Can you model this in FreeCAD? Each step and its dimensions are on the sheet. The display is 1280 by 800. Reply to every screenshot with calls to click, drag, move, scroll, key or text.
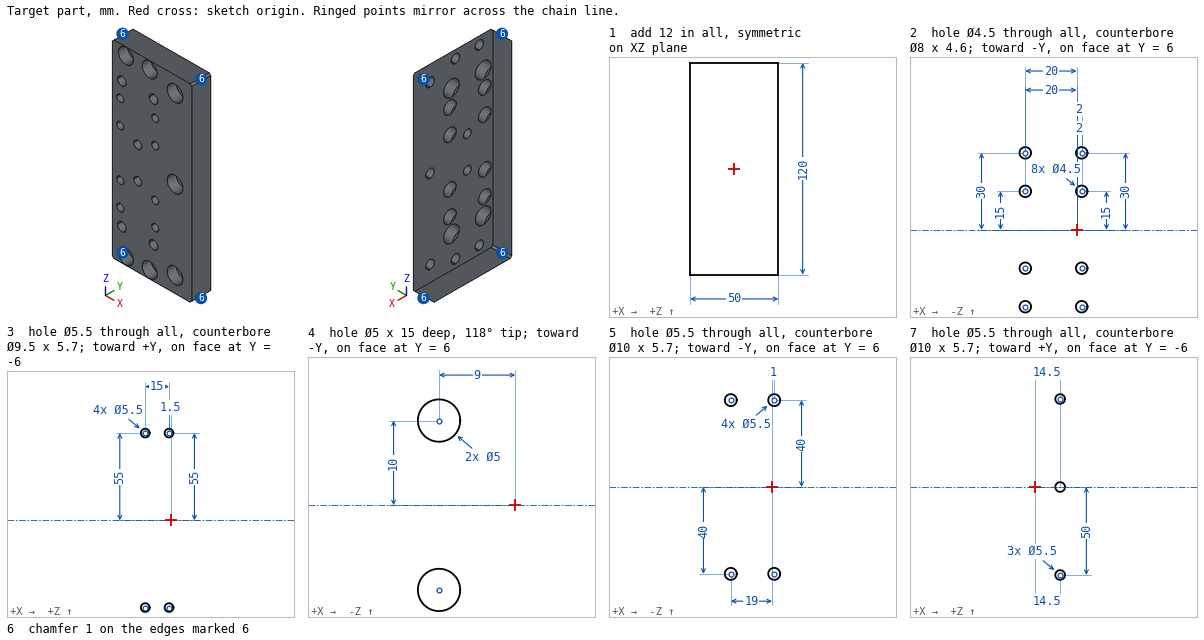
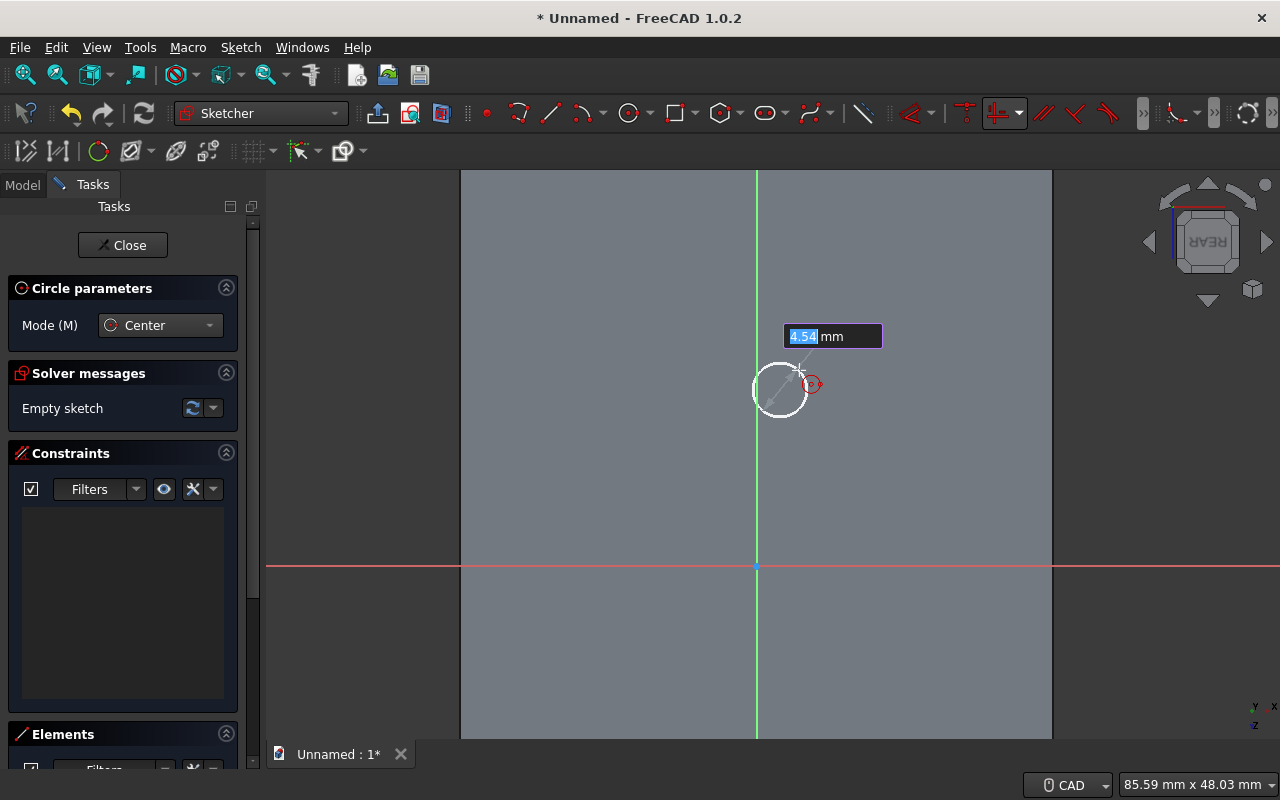
text(4.5)
key(Return)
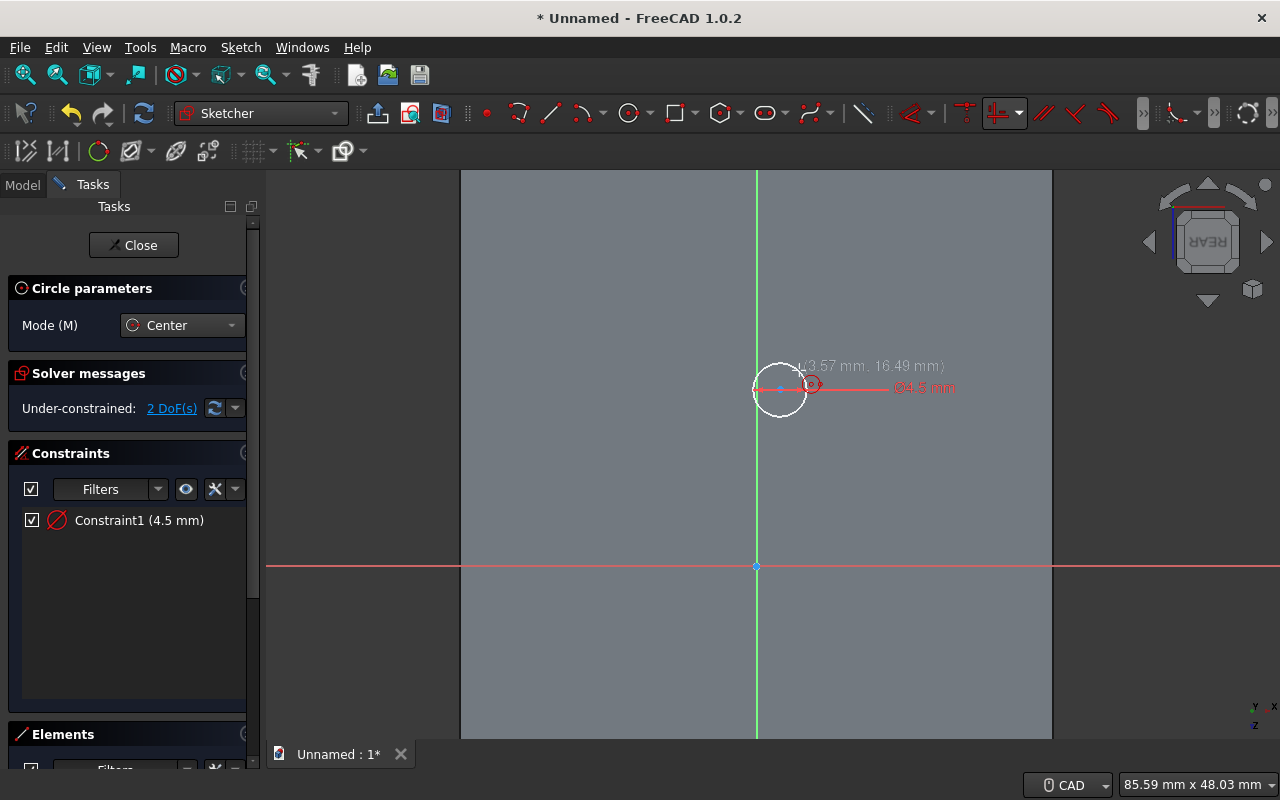
click(520, 211)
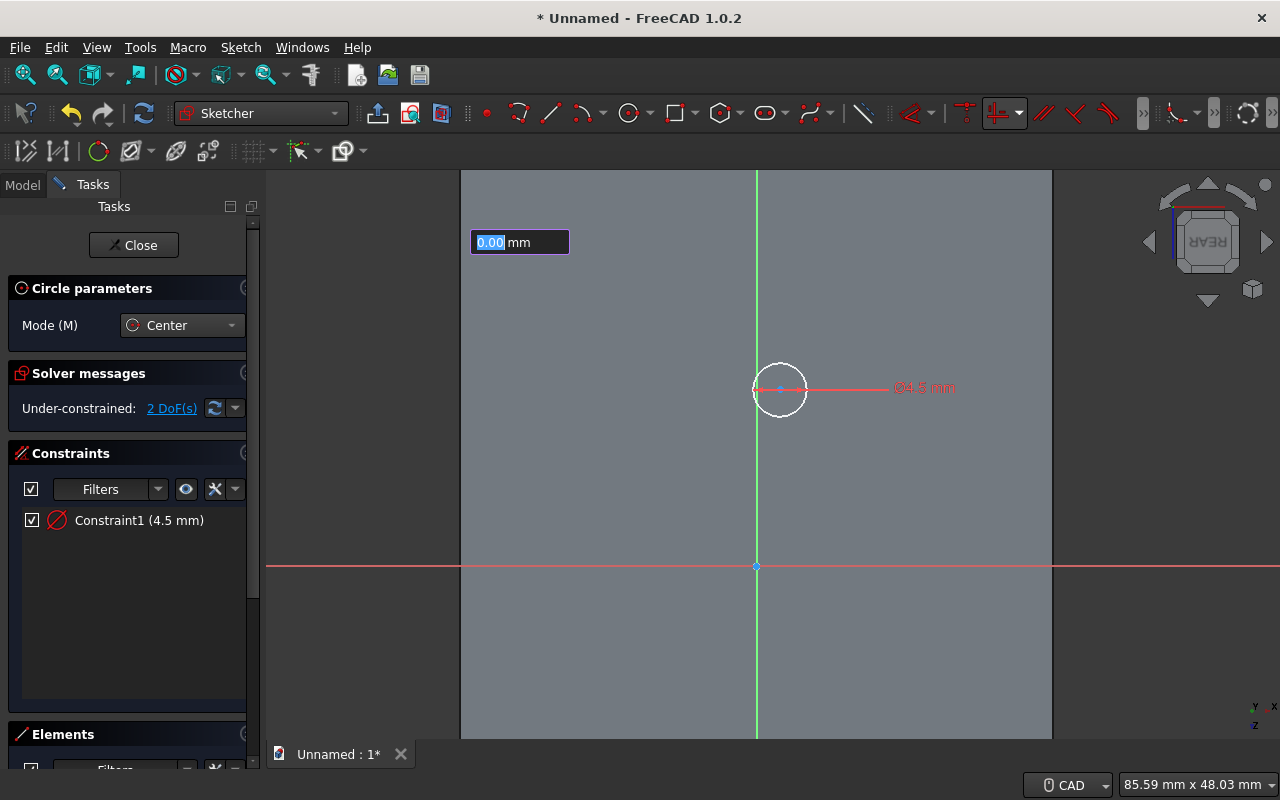
scroll(749, 363, down, 4)
move(655, 286)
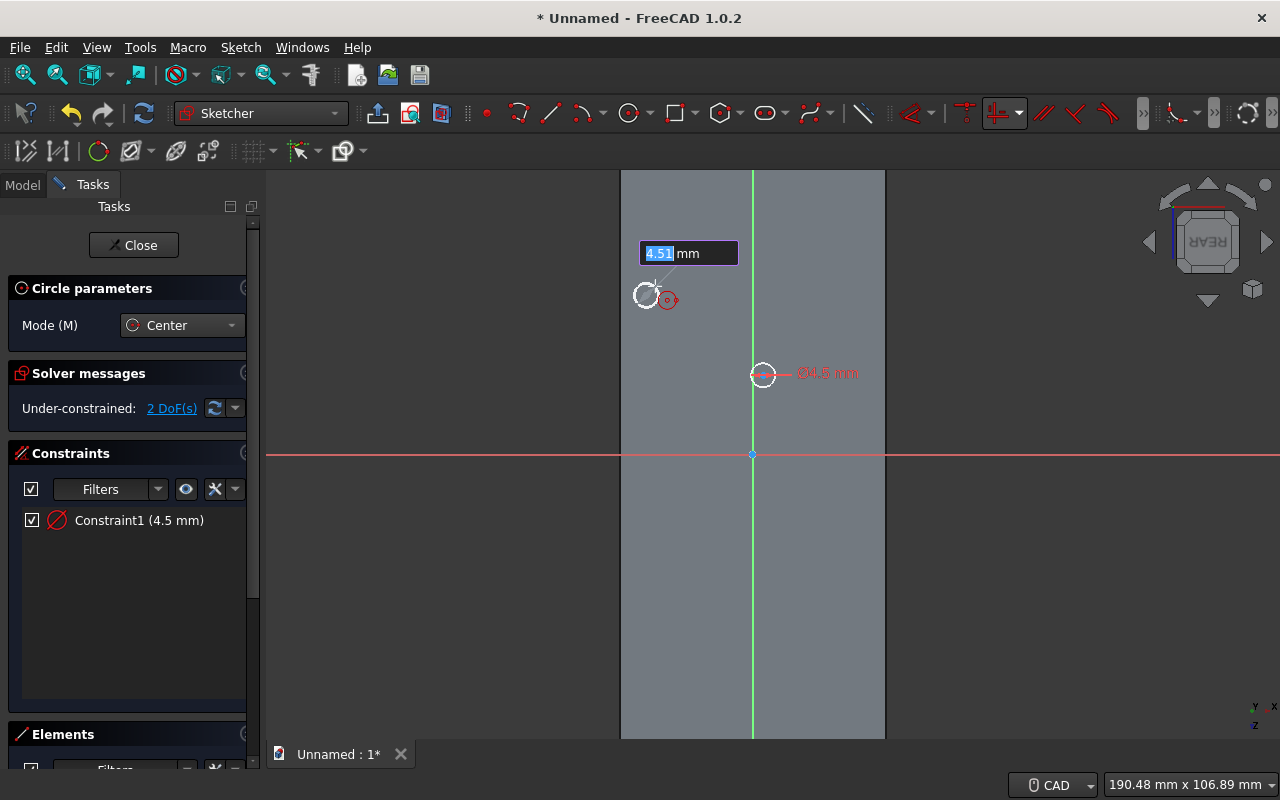
text(4.5)
key(Return)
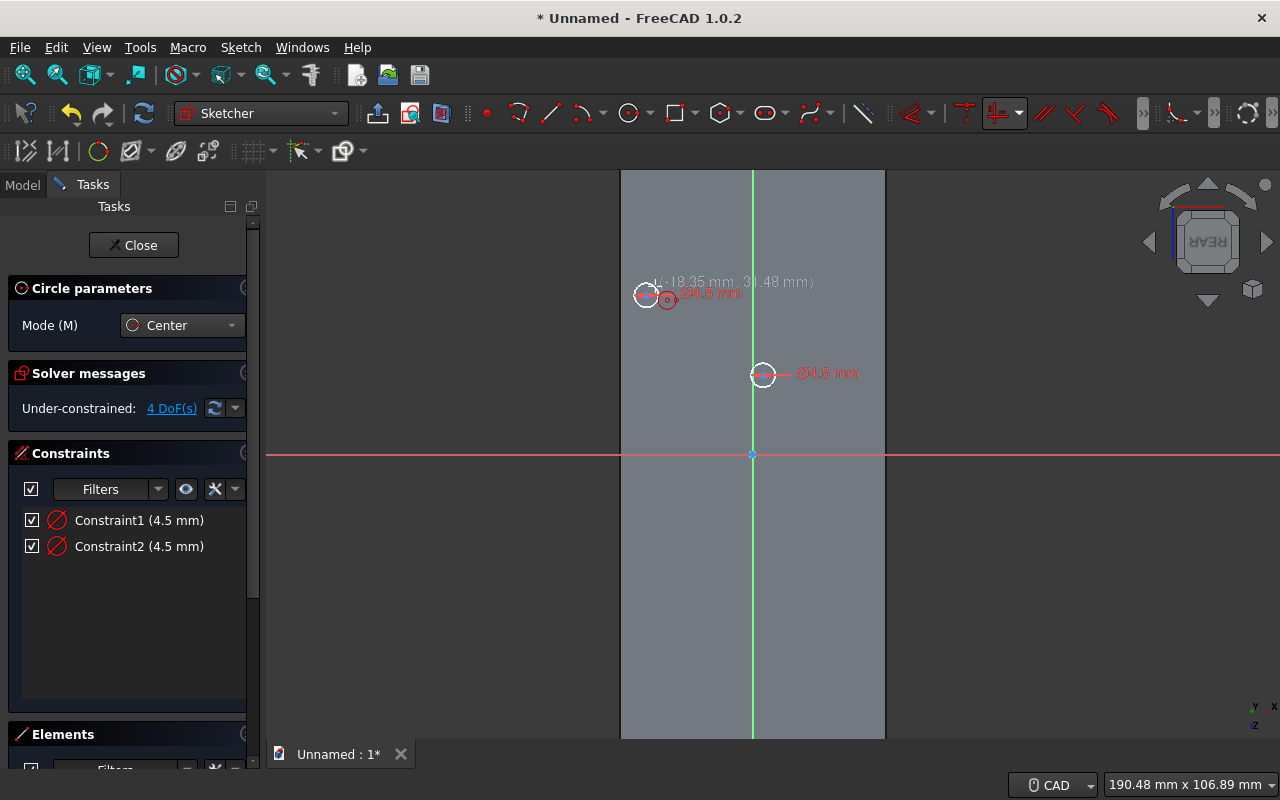
scroll(763, 295, up, 4)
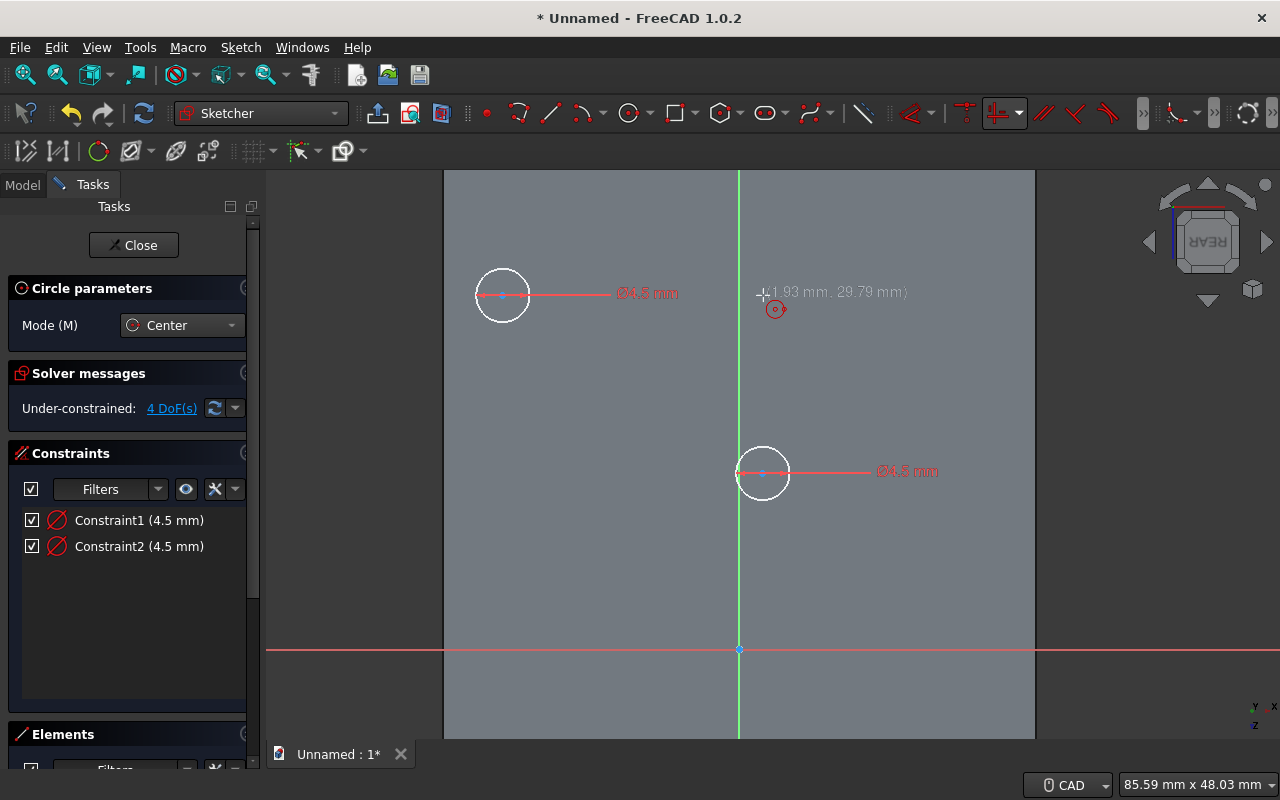
click(763, 294)
move(782, 276)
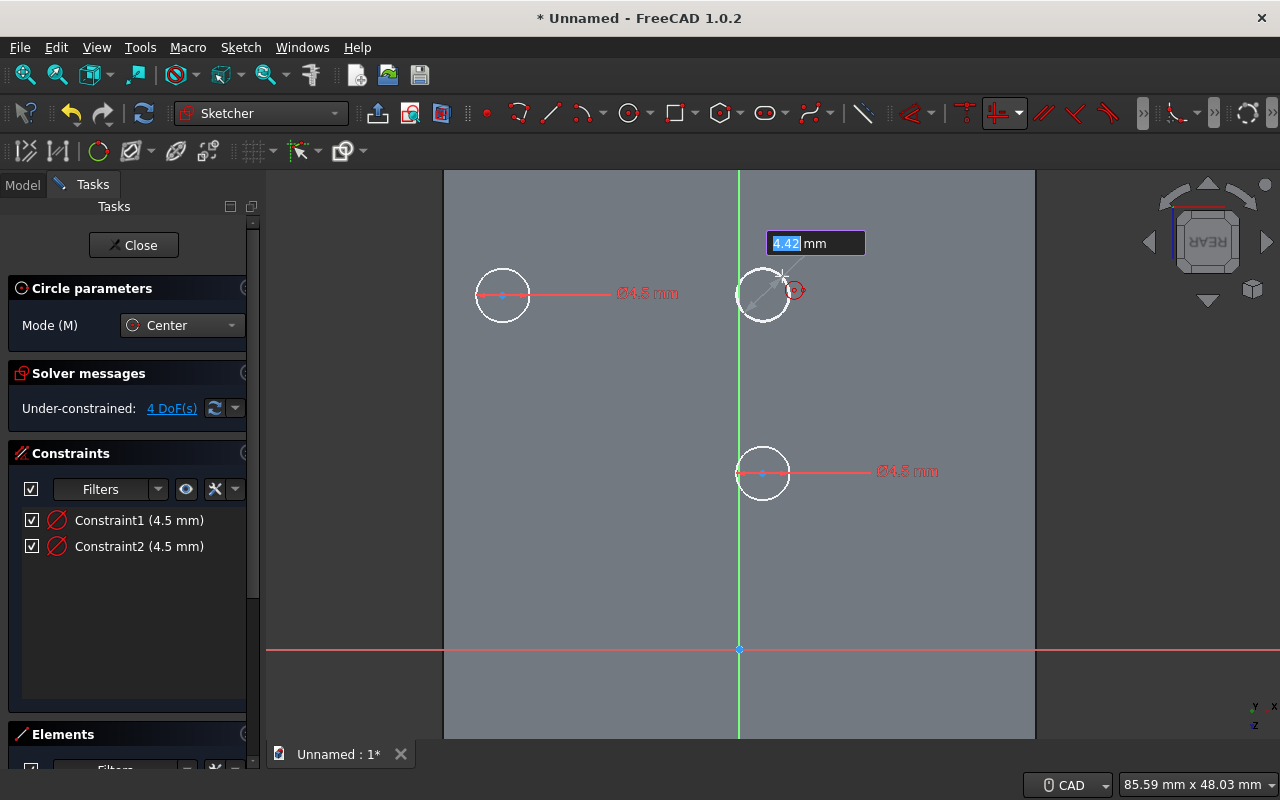
text(4.5)
key(Return)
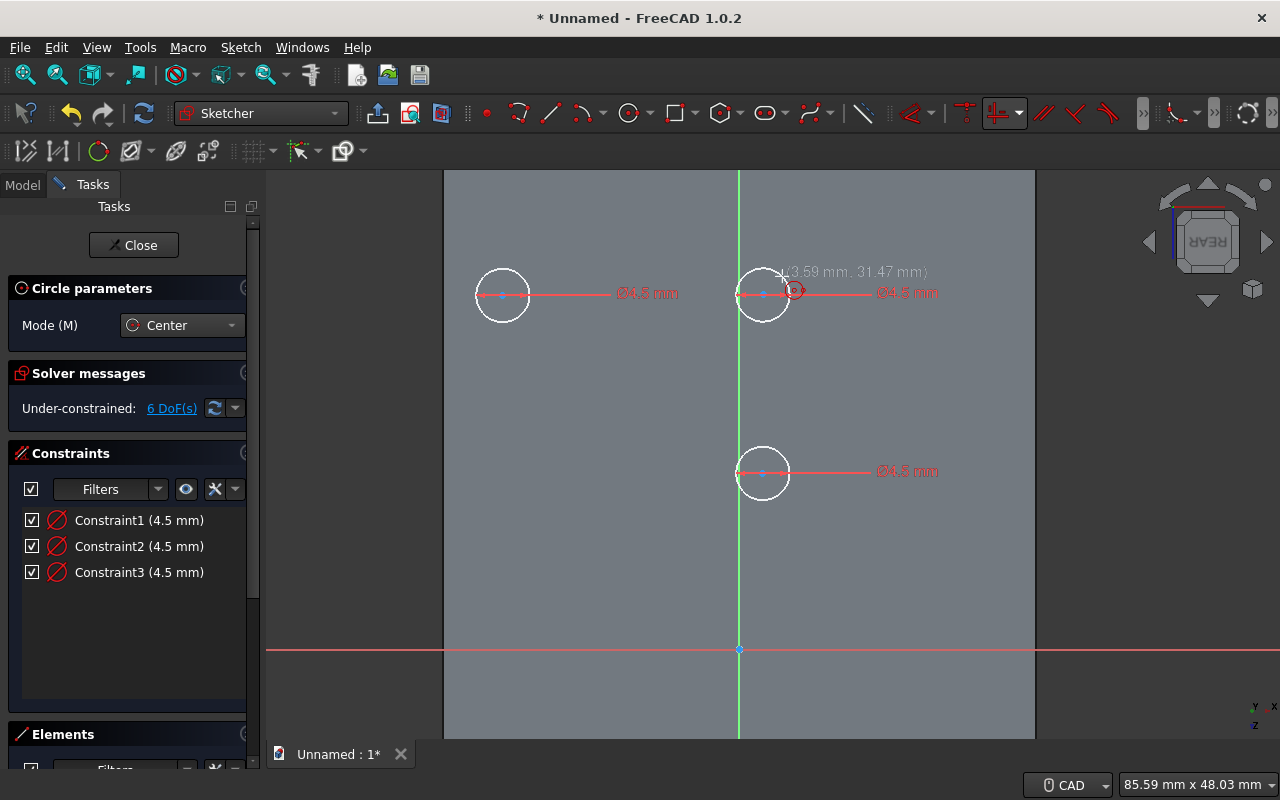
click(503, 472)
move(521, 453)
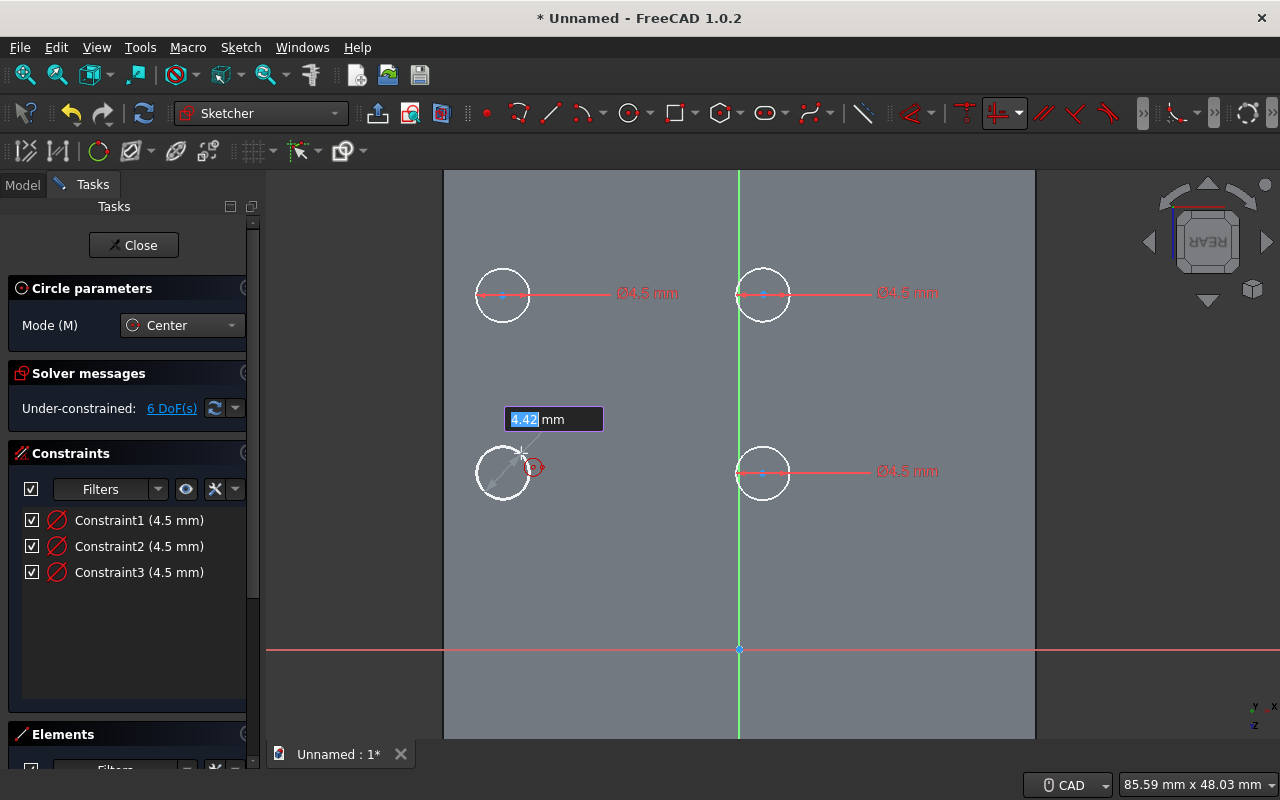
text(4.5)
key(Return)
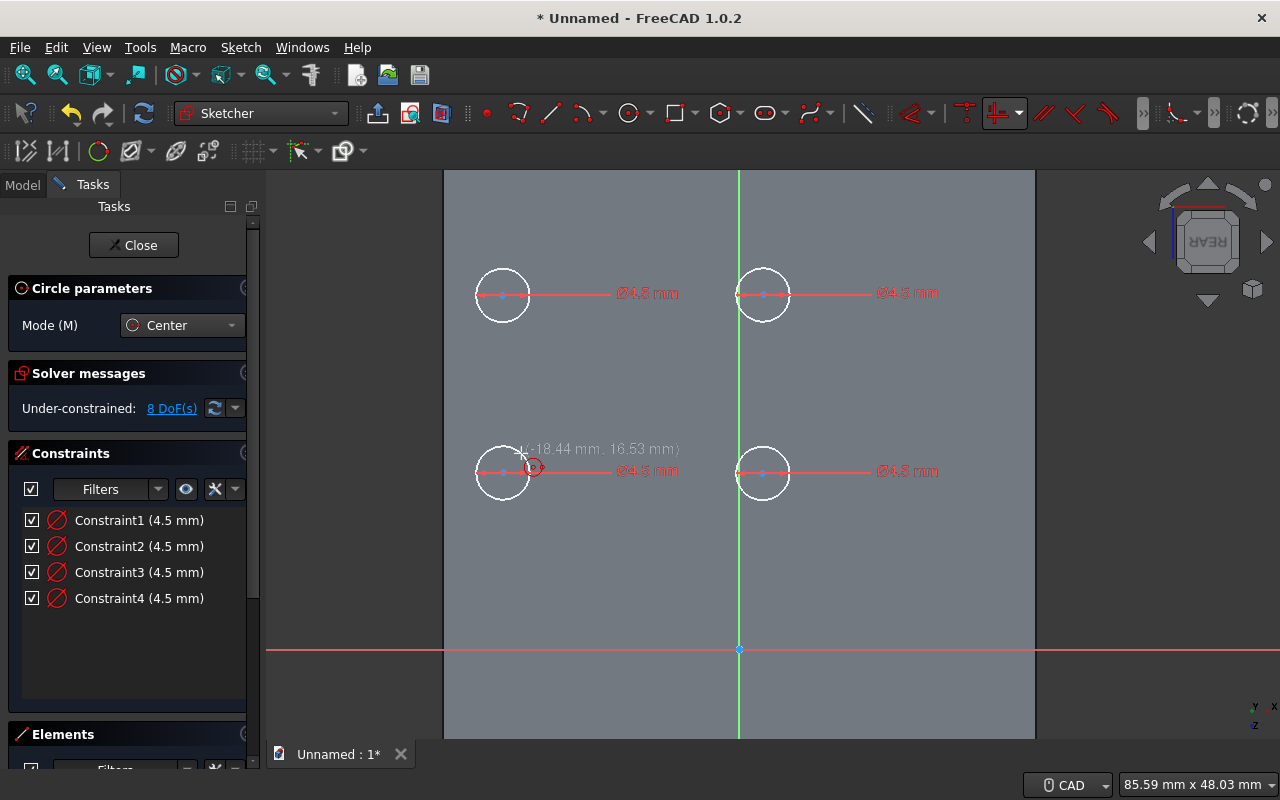
scroll(763, 295, down, 4)